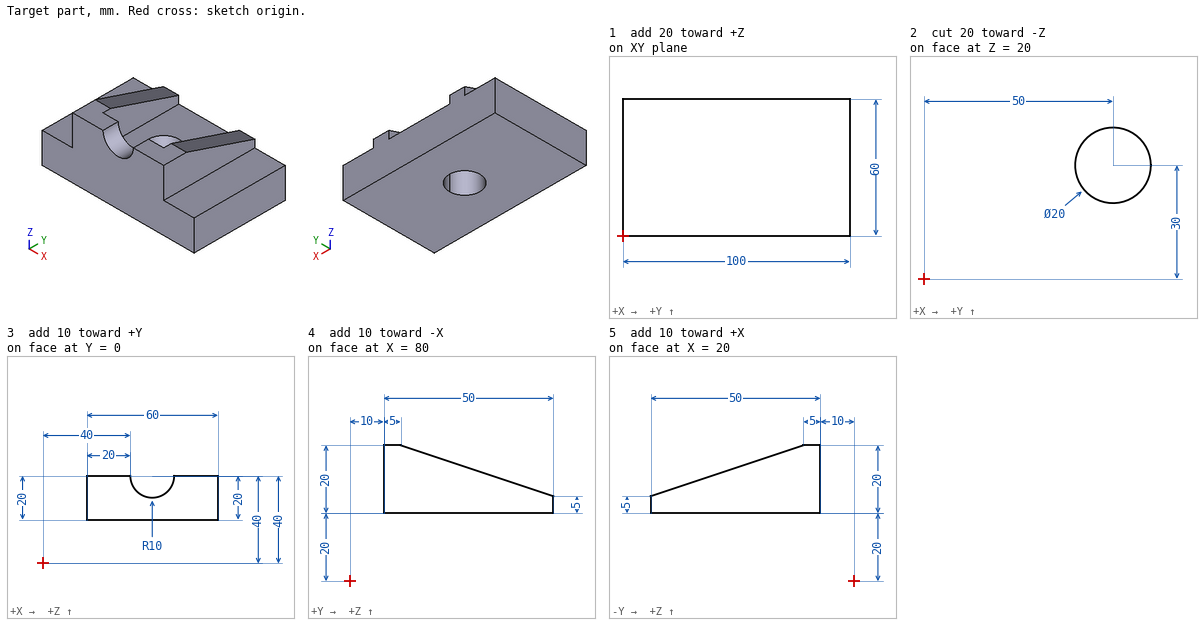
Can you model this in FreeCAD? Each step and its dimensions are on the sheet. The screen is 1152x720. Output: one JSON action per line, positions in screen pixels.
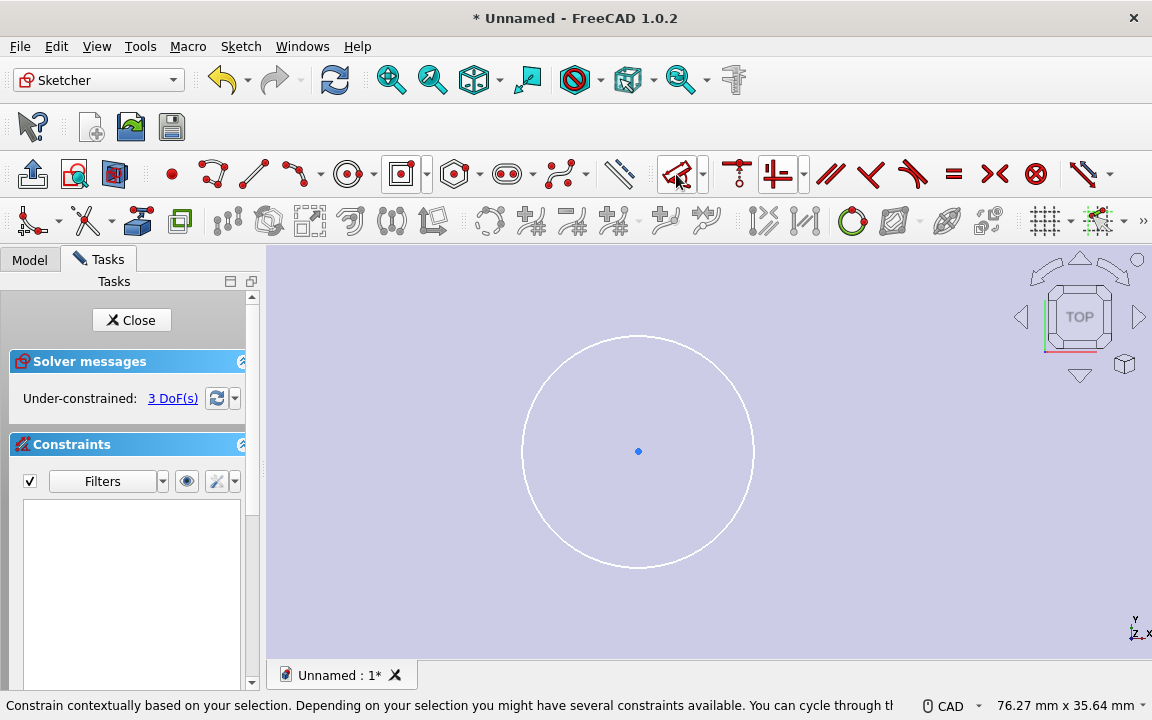
{"action": "left_click", "coordinate": [720, 370]}
{"action": "left_click", "coordinate": [743, 347]}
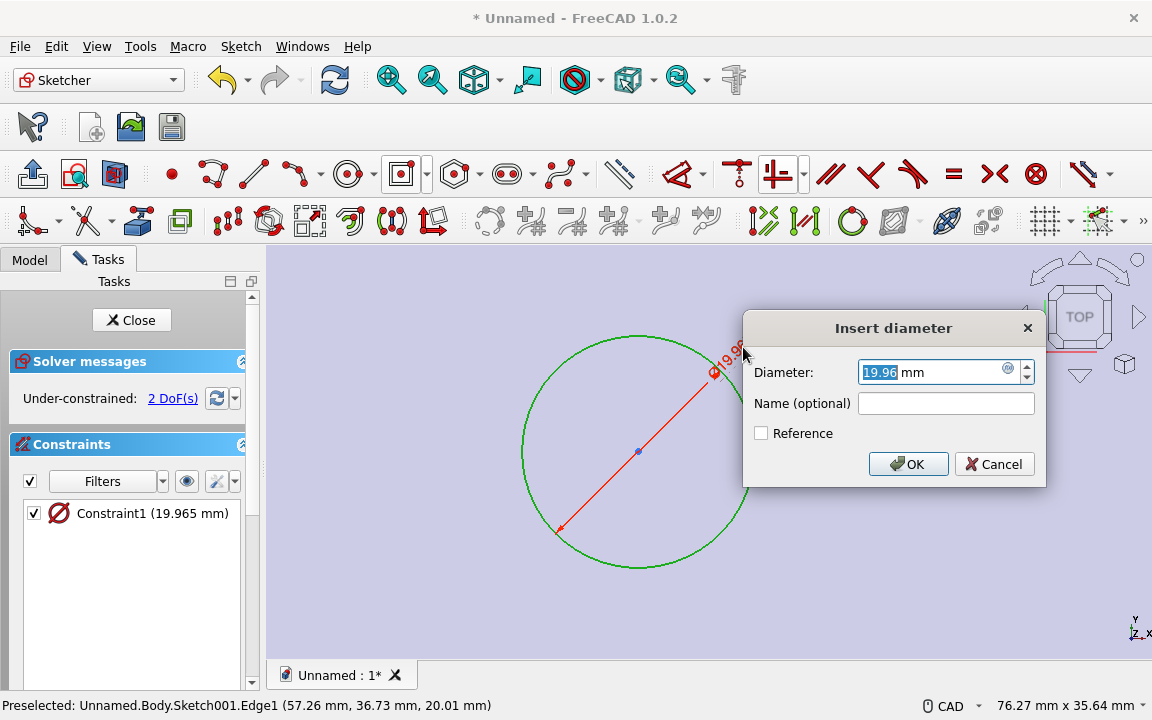
{"action": "type", "text": "20"}
{"action": "key", "text": "Return"}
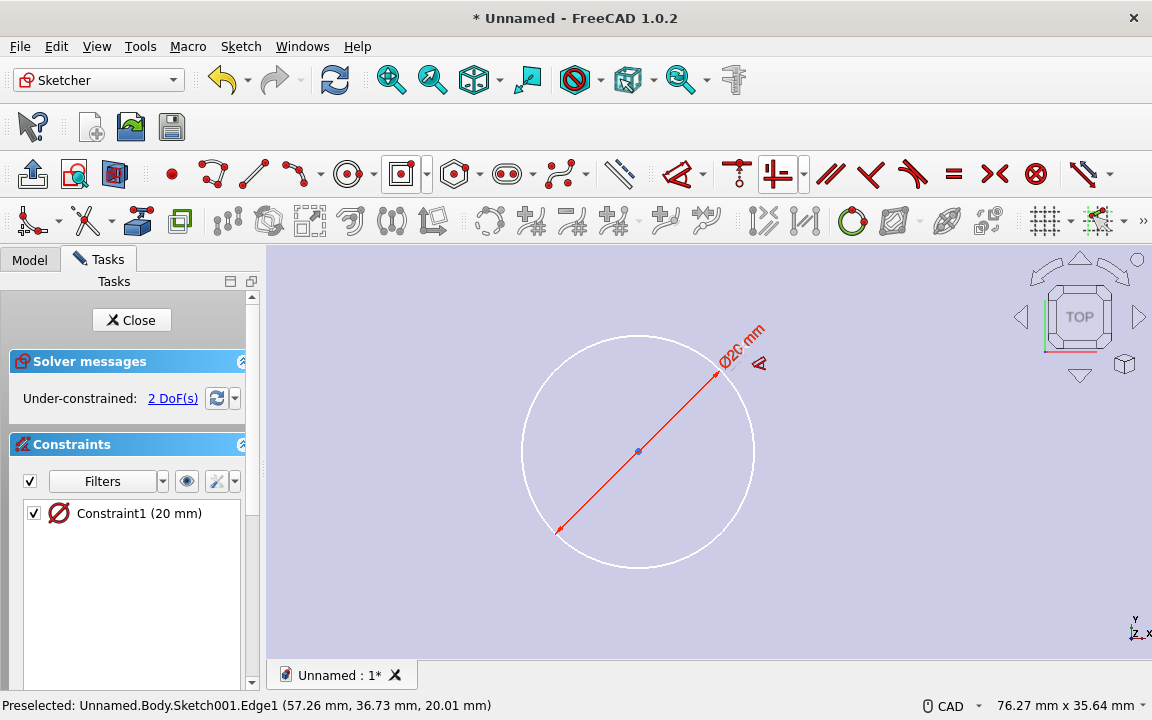
{"action": "left_click", "coordinate": [638, 452]}
{"action": "left_click", "coordinate": [466, 418]}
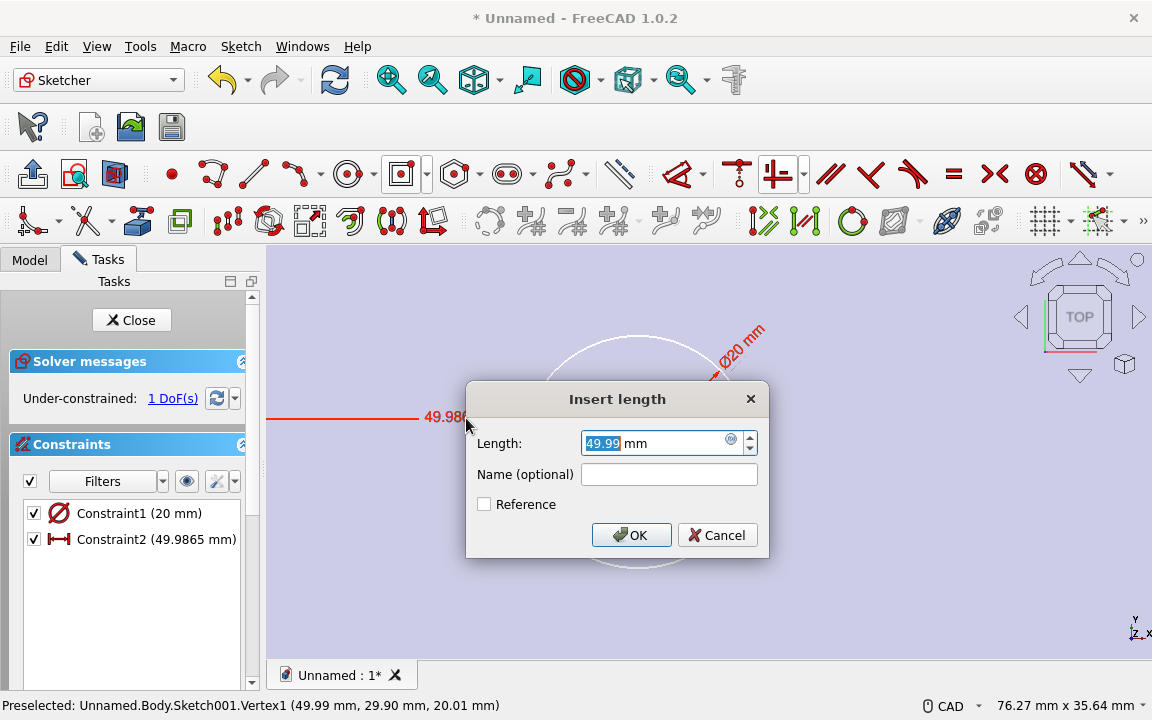
{"action": "type", "text": "50"}
{"action": "key", "text": "Return"}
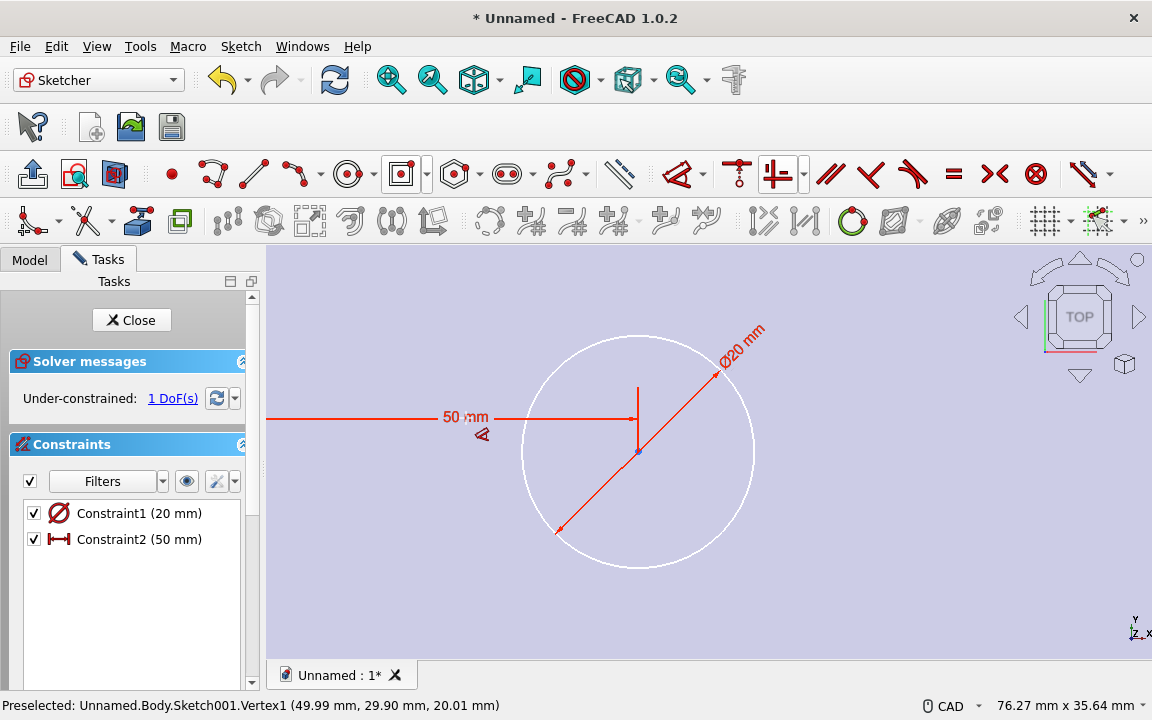
{"action": "left_click", "coordinate": [638, 452]}
{"action": "left_click", "coordinate": [672, 541]}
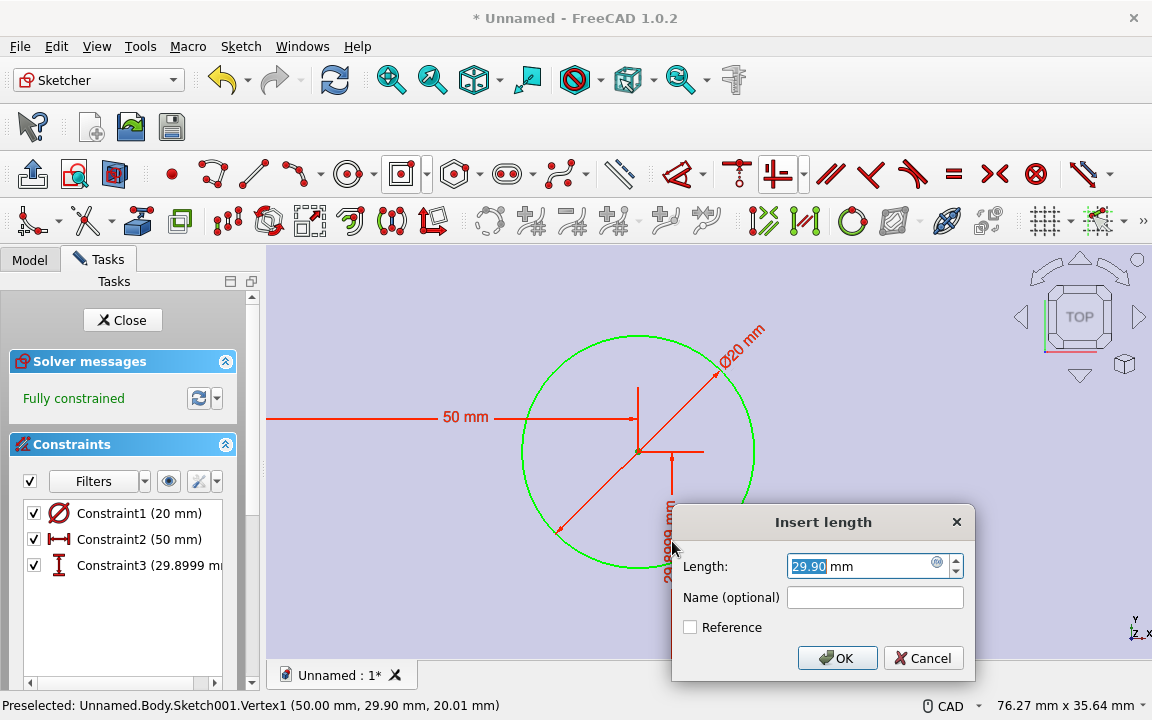
{"action": "type", "text": "30"}
{"action": "key", "text": "Return"}
{"action": "key", "text": "Escape"}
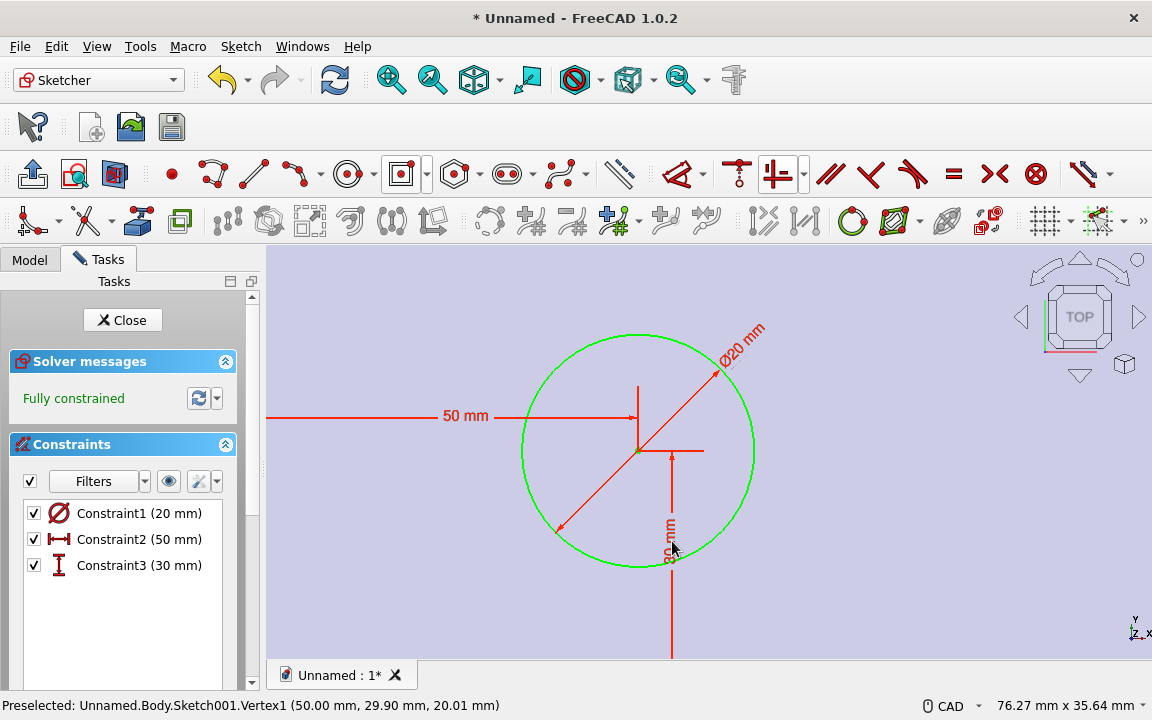
{"action": "left_click", "coordinate": [123, 320]}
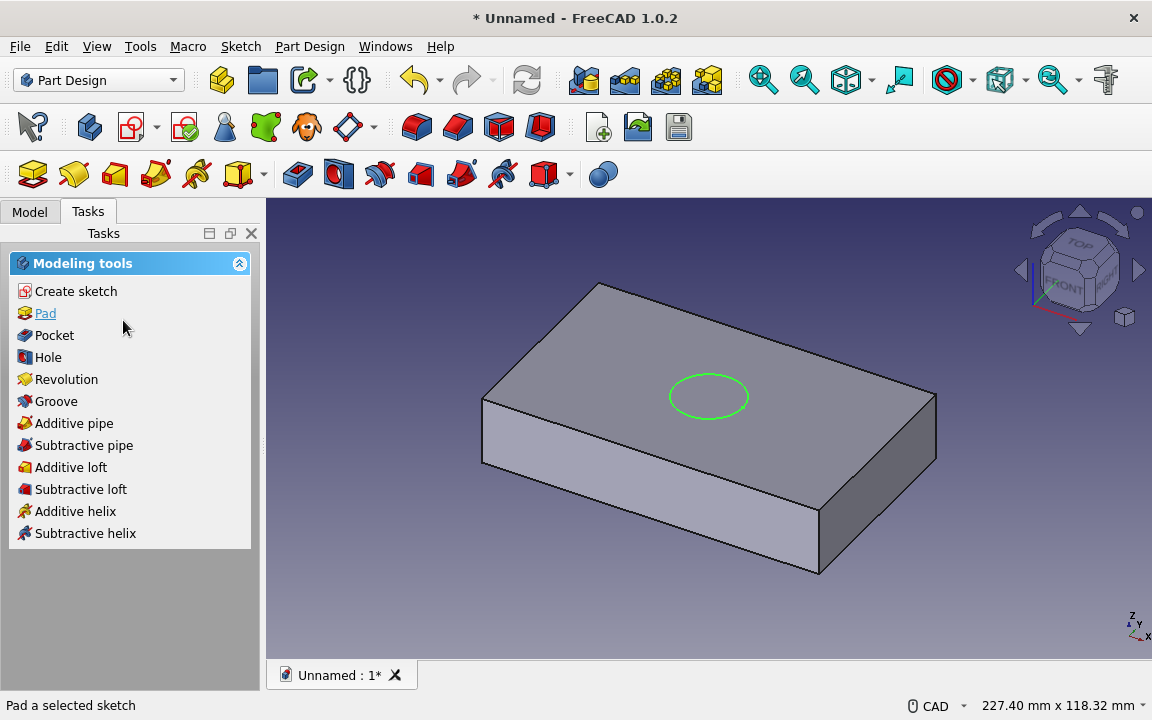
{"action": "left_click", "coordinate": [298, 174]}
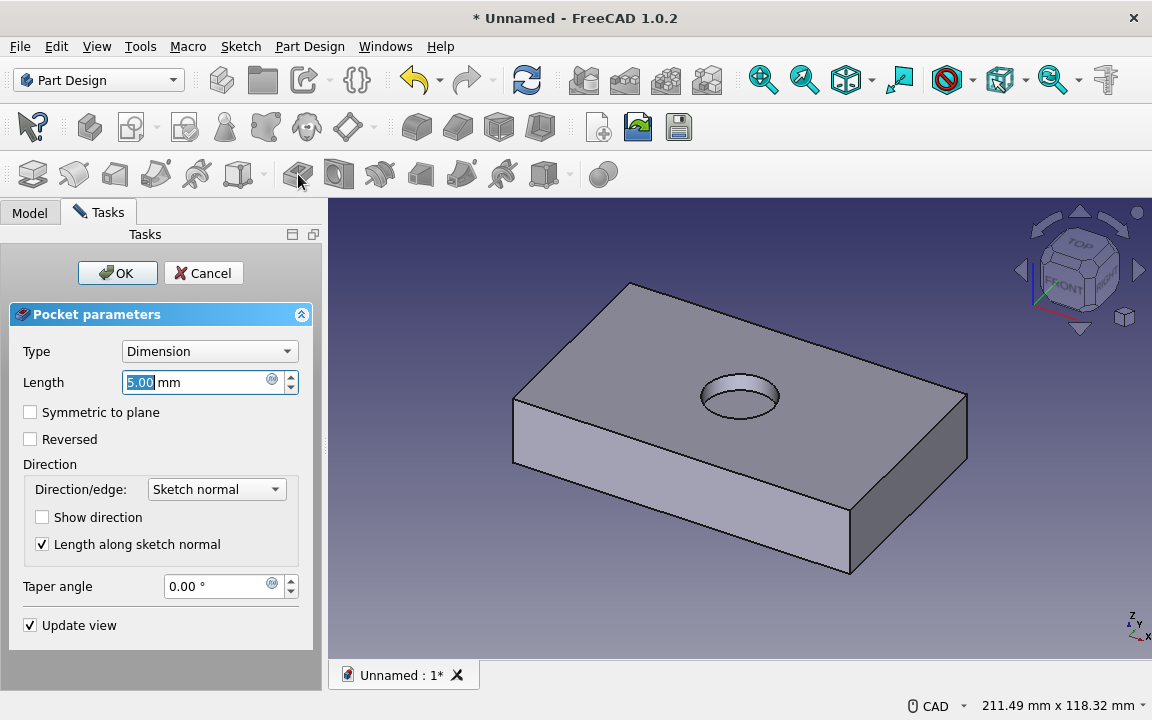
{"action": "type", "text": "20"}
{"action": "key", "text": "Tab"}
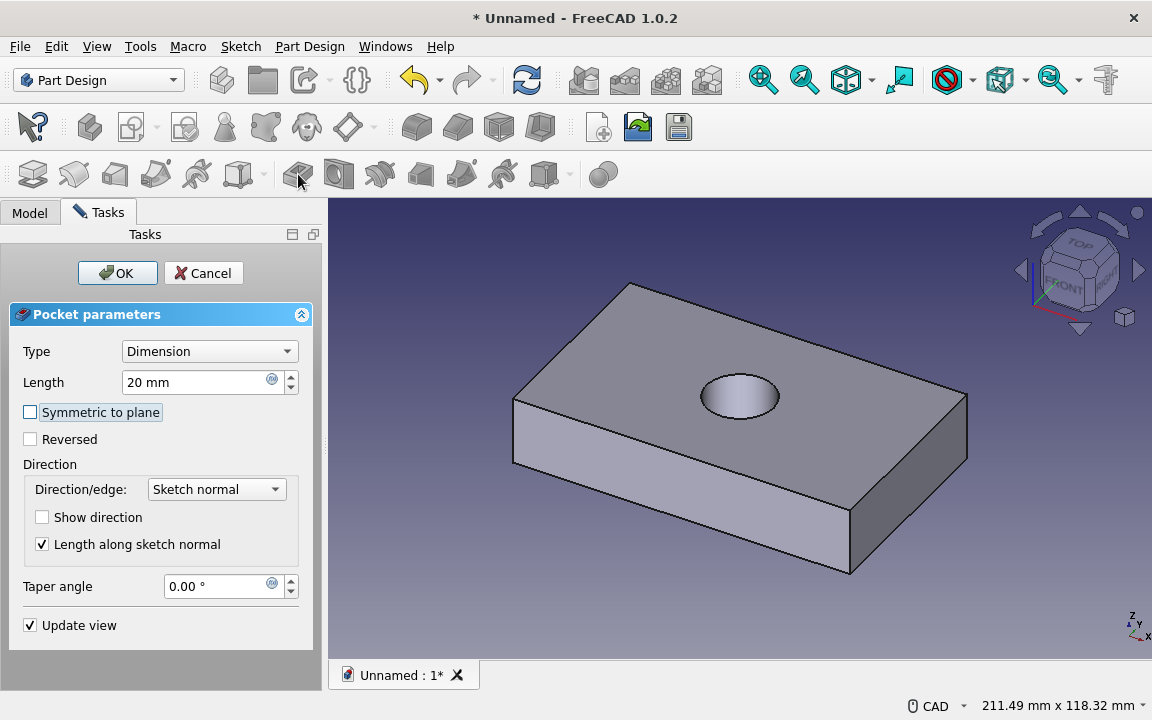
{"action": "left_click", "coordinate": [118, 273]}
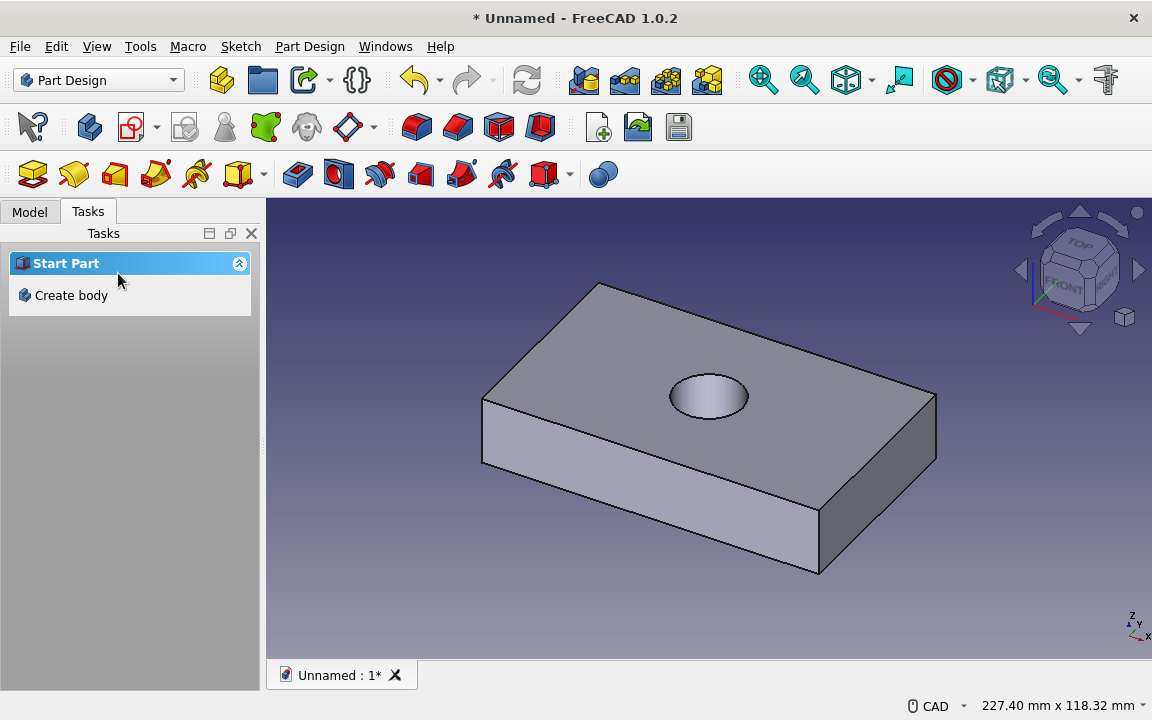
{"action": "left_click", "coordinate": [747, 517]}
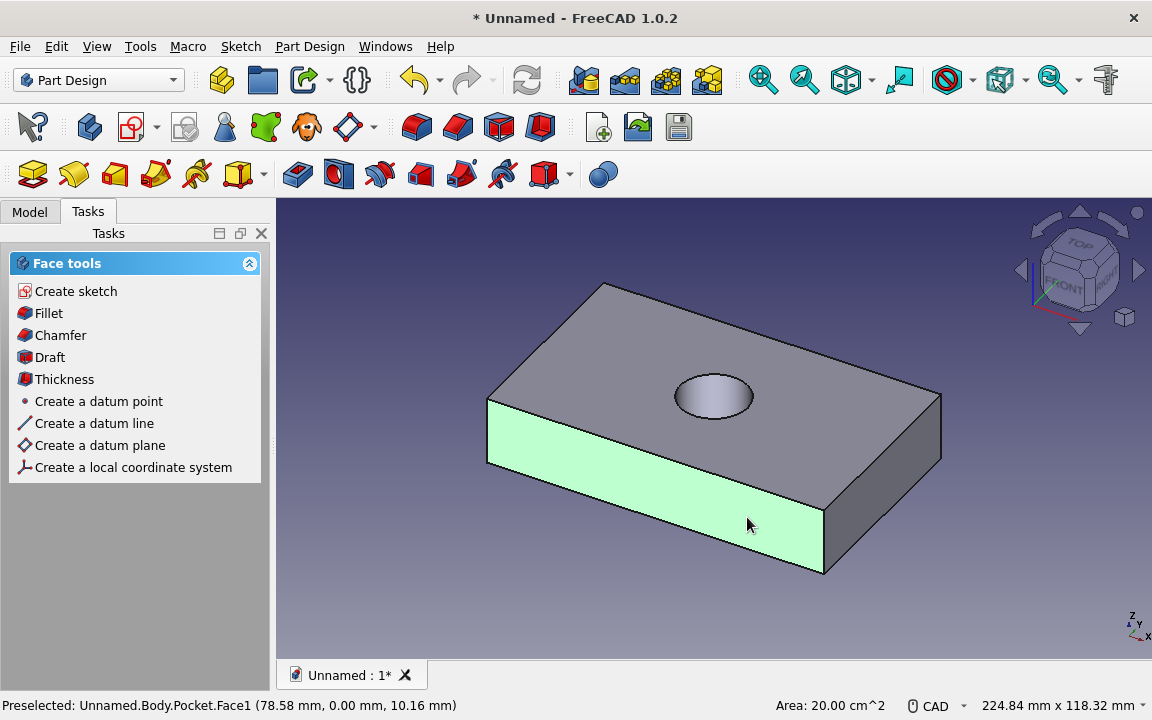
{"action": "left_click", "coordinate": [130, 128]}